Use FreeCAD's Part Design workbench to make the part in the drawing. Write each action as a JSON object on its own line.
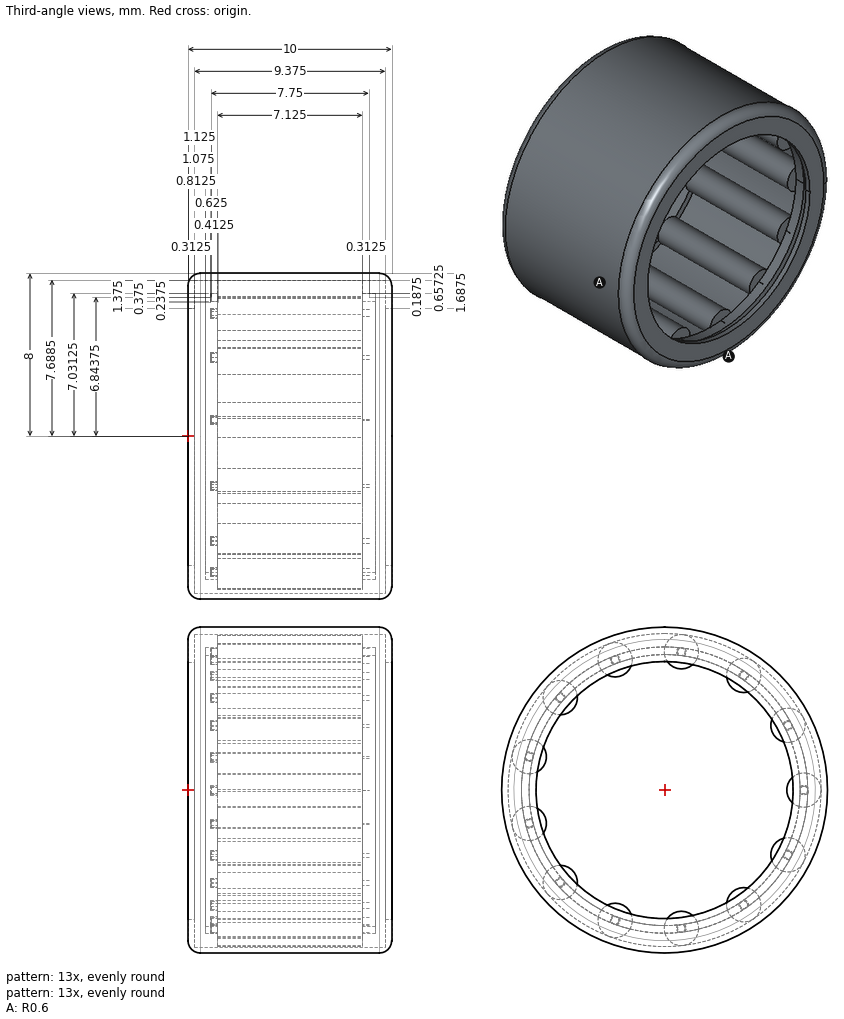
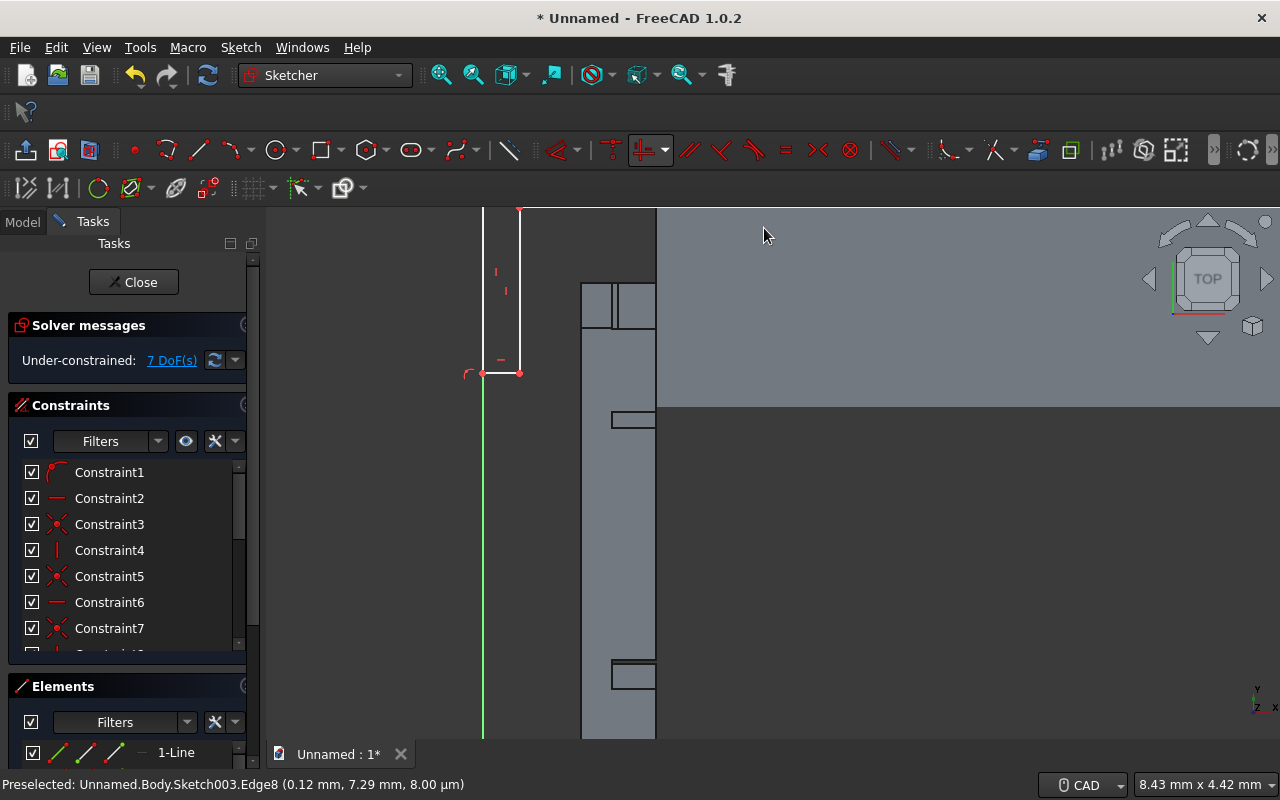
{"action": "left_click", "coordinate": [556, 150]}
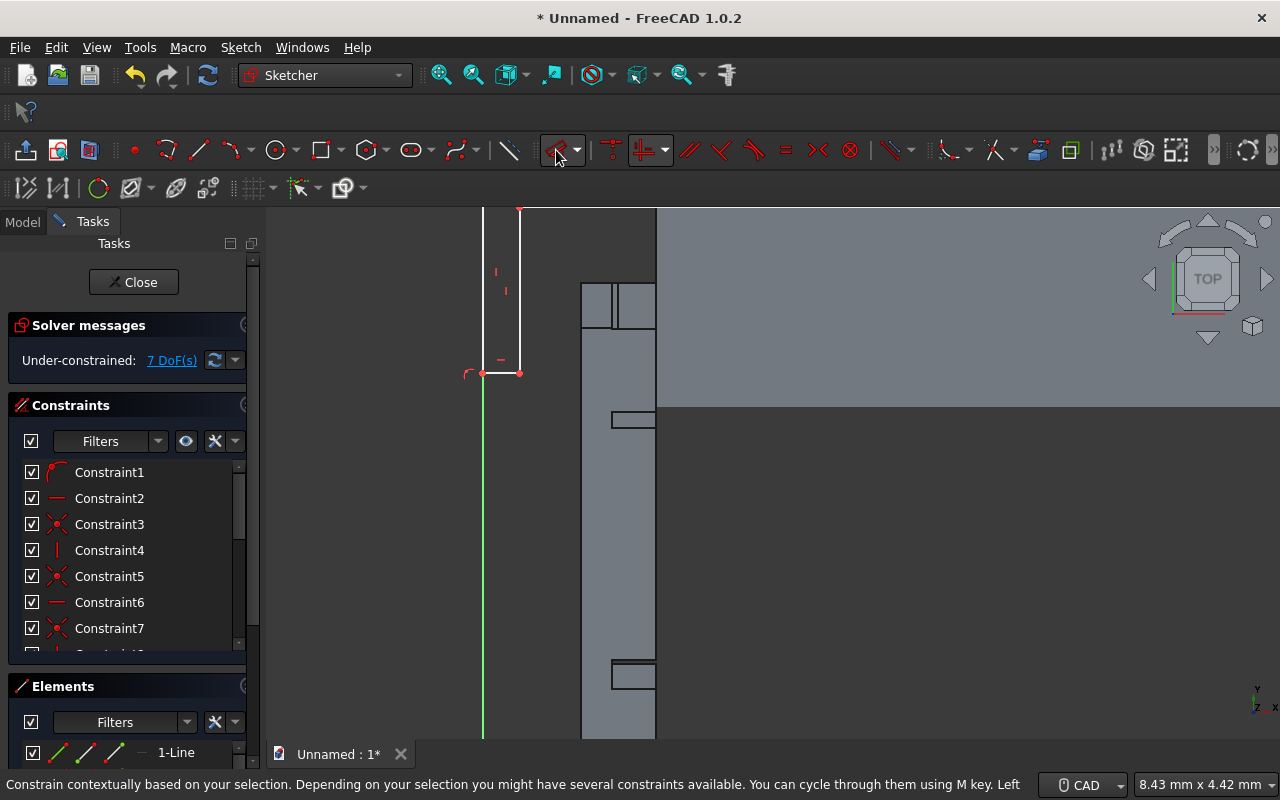
{"action": "scroll", "coordinate": [483, 371], "scroll_direction": "down", "scroll_amount": 5}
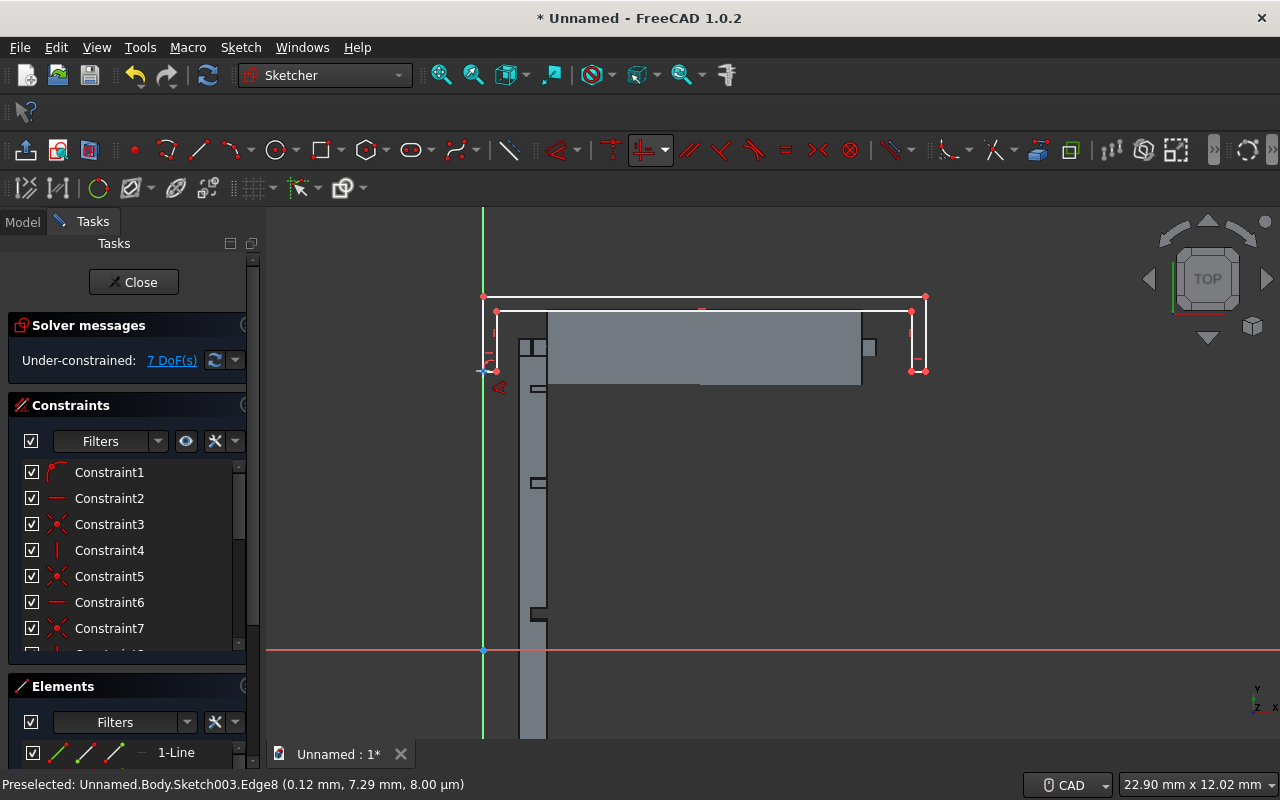
{"action": "left_click", "coordinate": [793, 297]}
{"action": "left_click", "coordinate": [704, 263]}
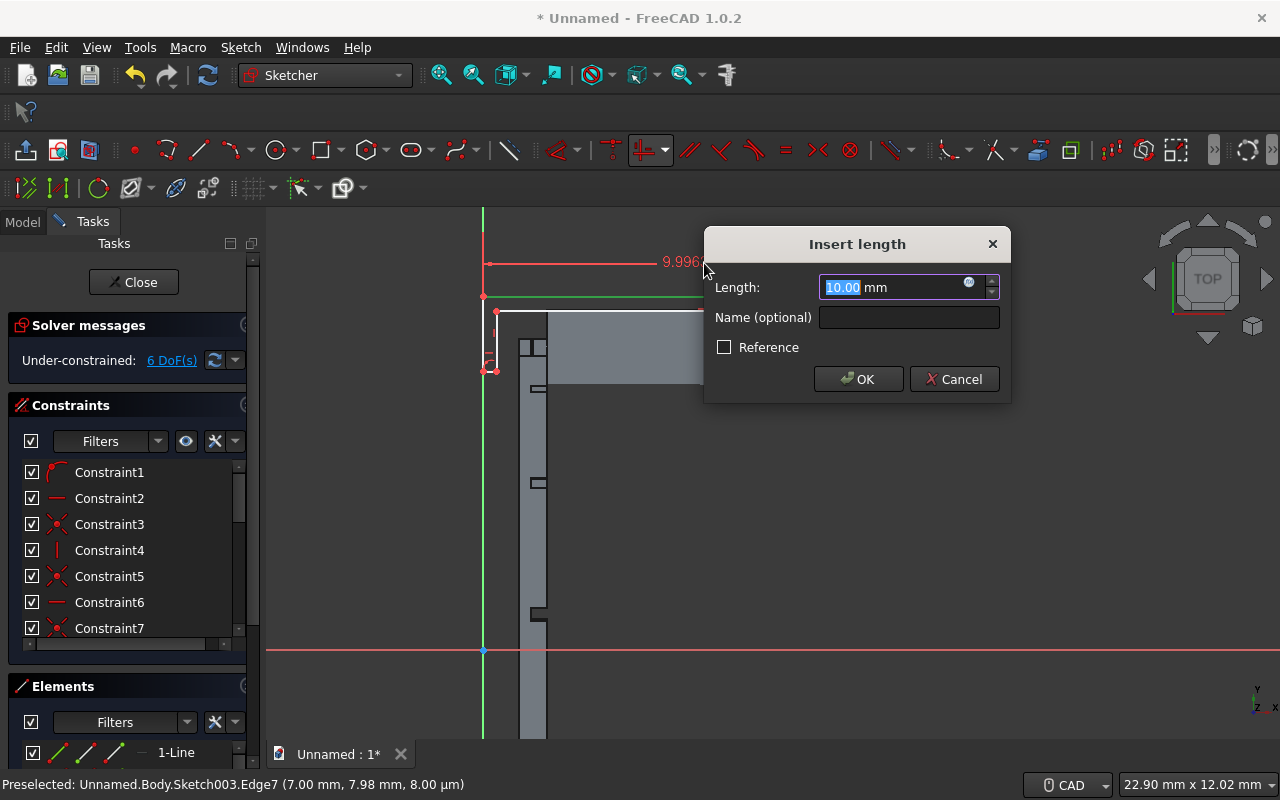
{"action": "type", "text": "10"}
{"action": "key", "text": "Return"}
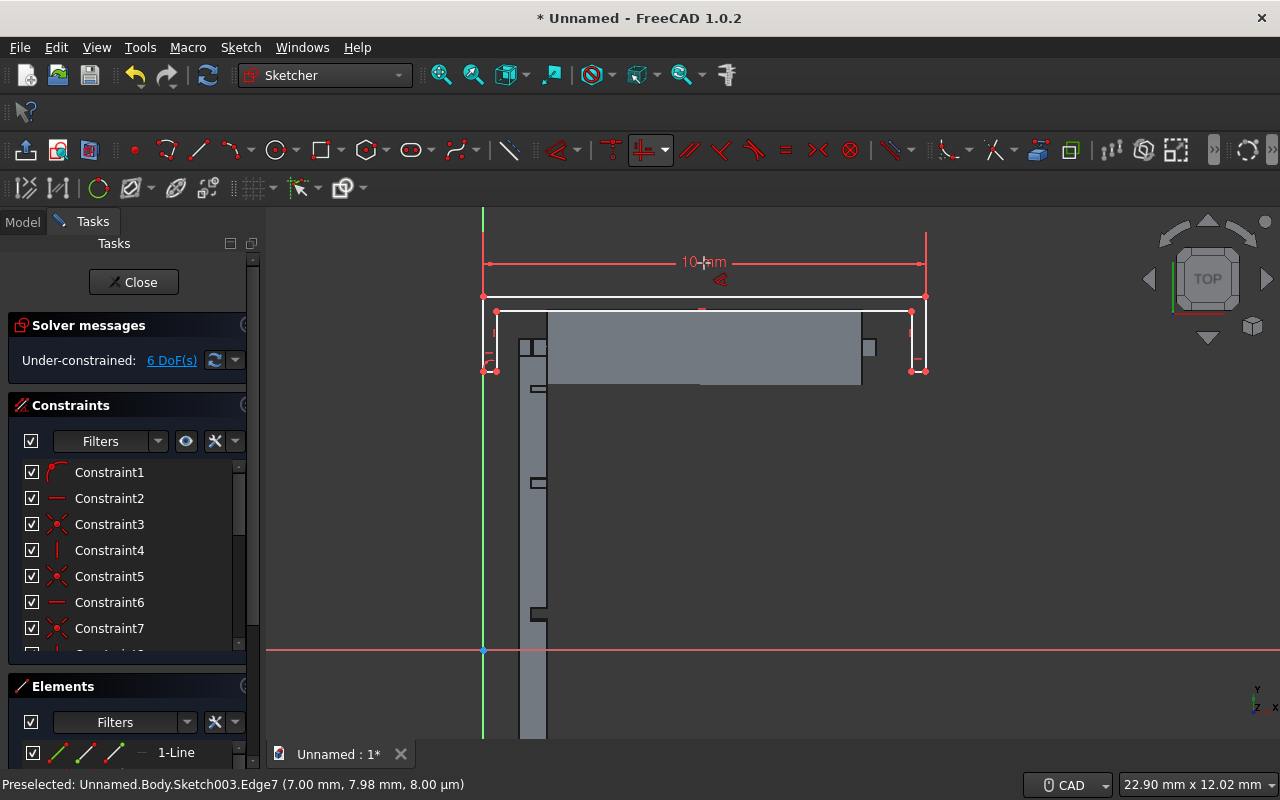
{"action": "left_click", "coordinate": [926, 297]}
{"action": "left_click", "coordinate": [960, 474]}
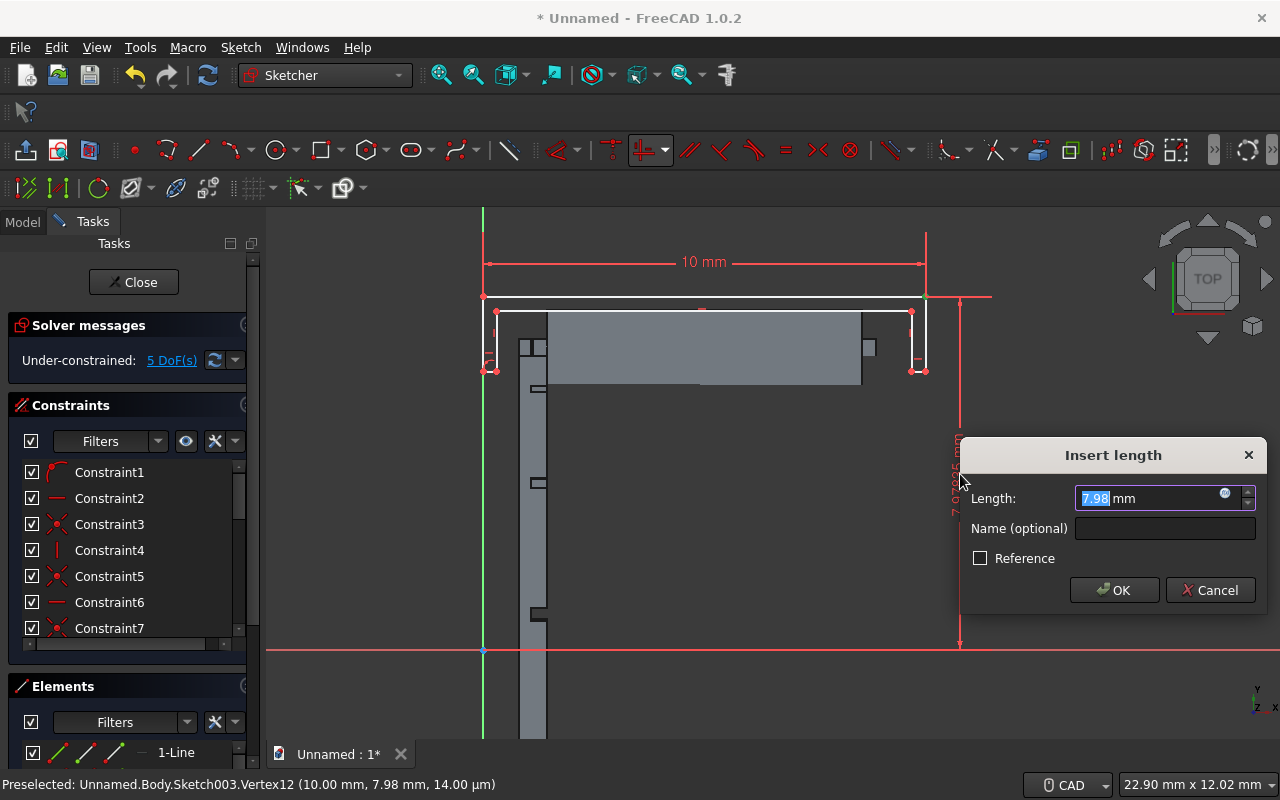
{"action": "type", "text": "8"}
{"action": "key", "text": "Return"}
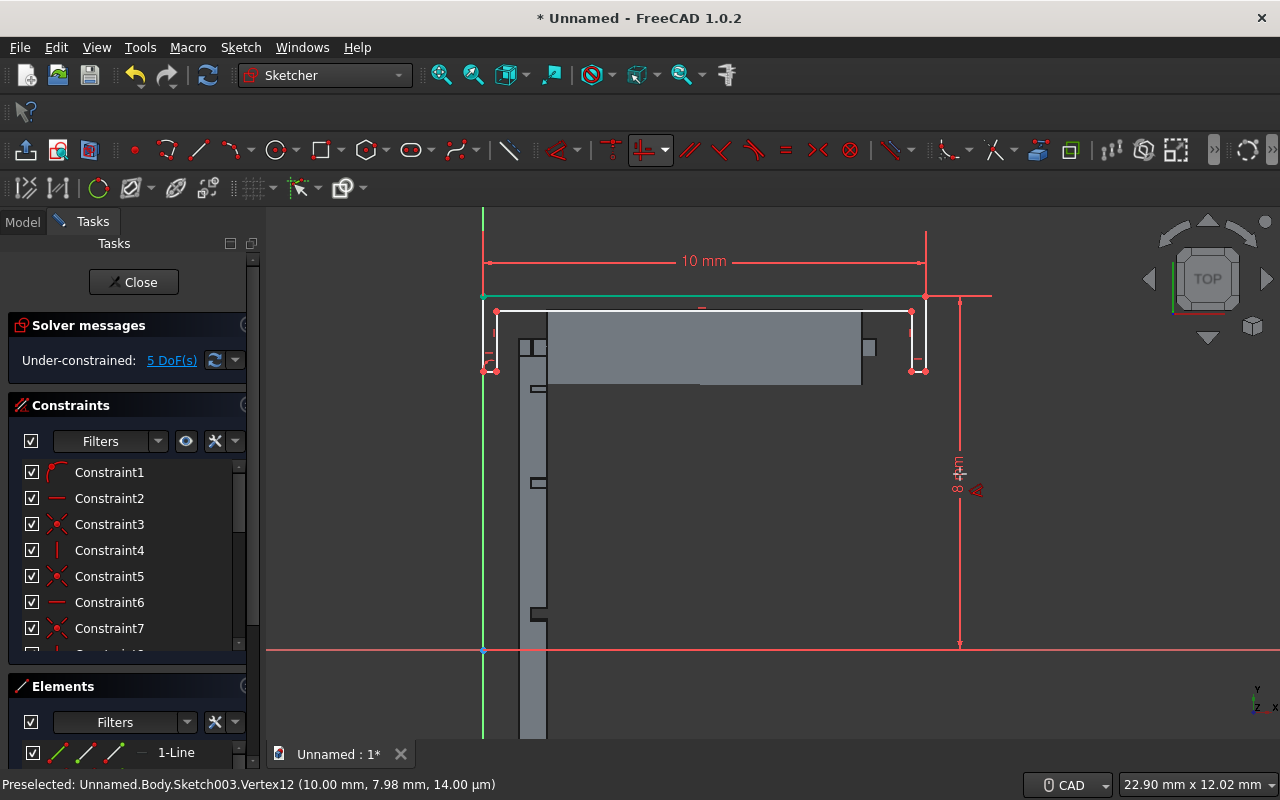
{"action": "left_click", "coordinate": [497, 354]}
{"action": "left_click", "coordinate": [463, 342]}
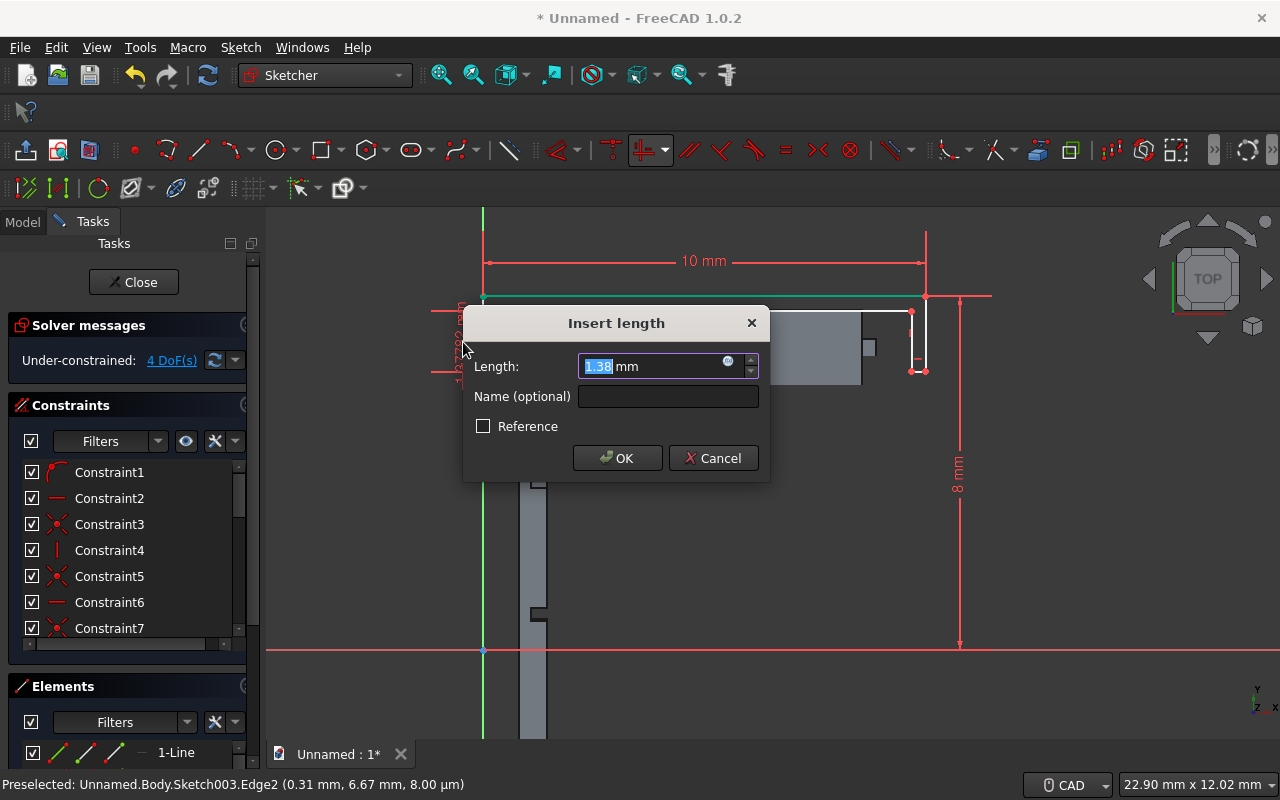
{"action": "type", "text": "1.375"}
{"action": "key", "text": "Return"}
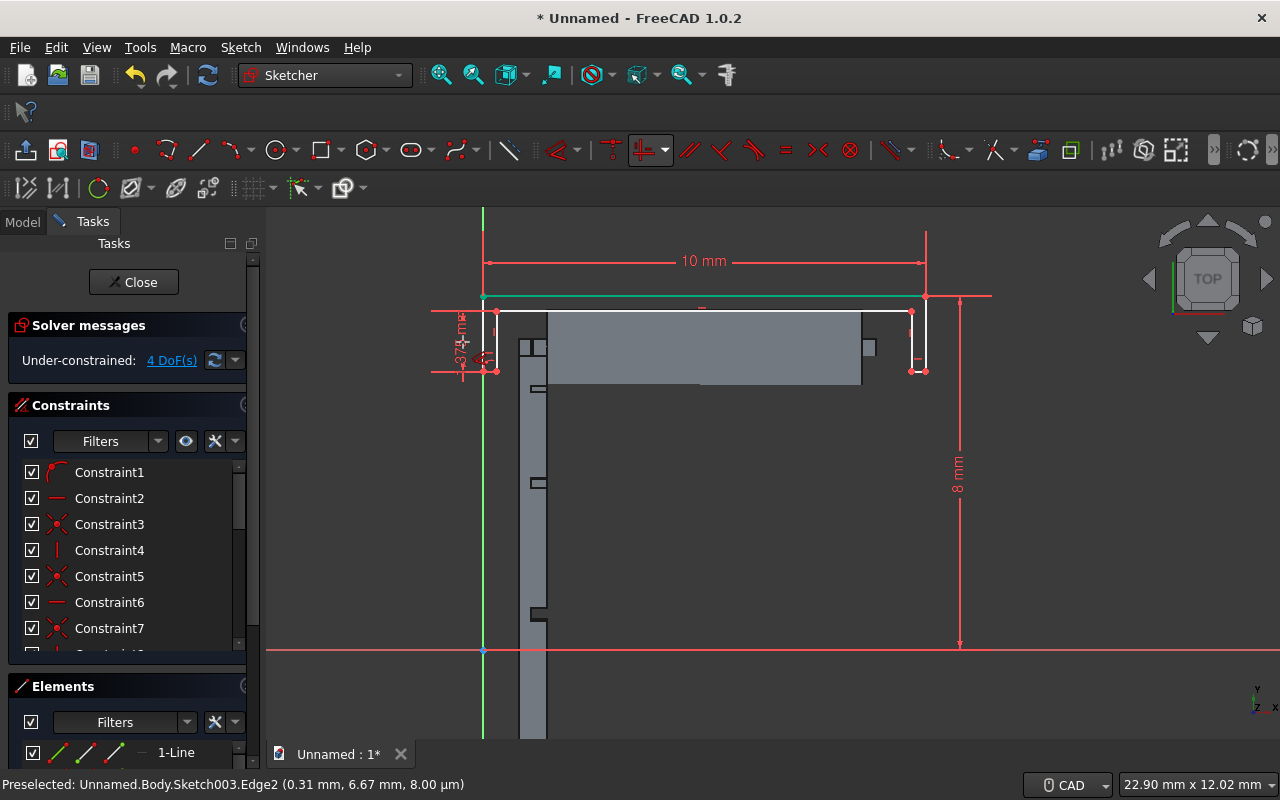
{"action": "left_click", "coordinate": [621, 311]}
{"action": "left_click", "coordinate": [609, 277]}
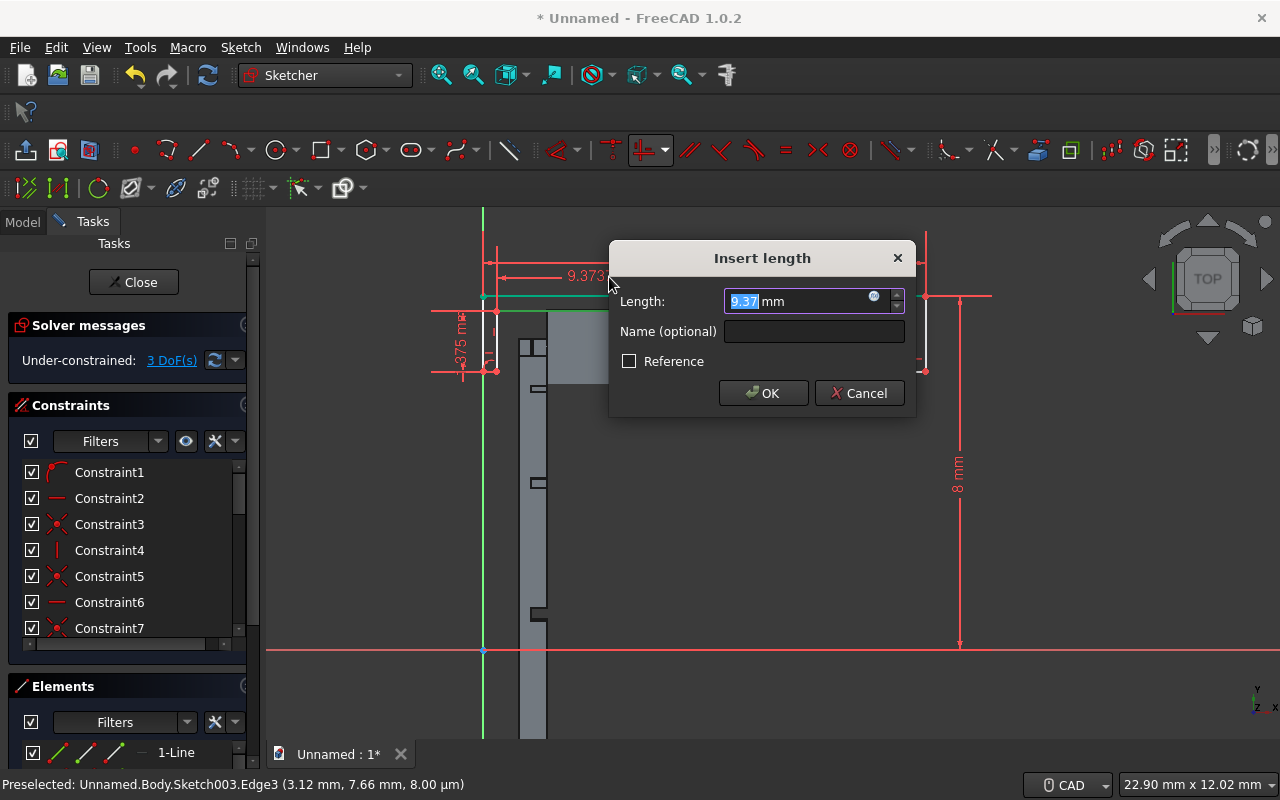
{"action": "type", "text": "9.375"}
{"action": "key", "text": "Return"}